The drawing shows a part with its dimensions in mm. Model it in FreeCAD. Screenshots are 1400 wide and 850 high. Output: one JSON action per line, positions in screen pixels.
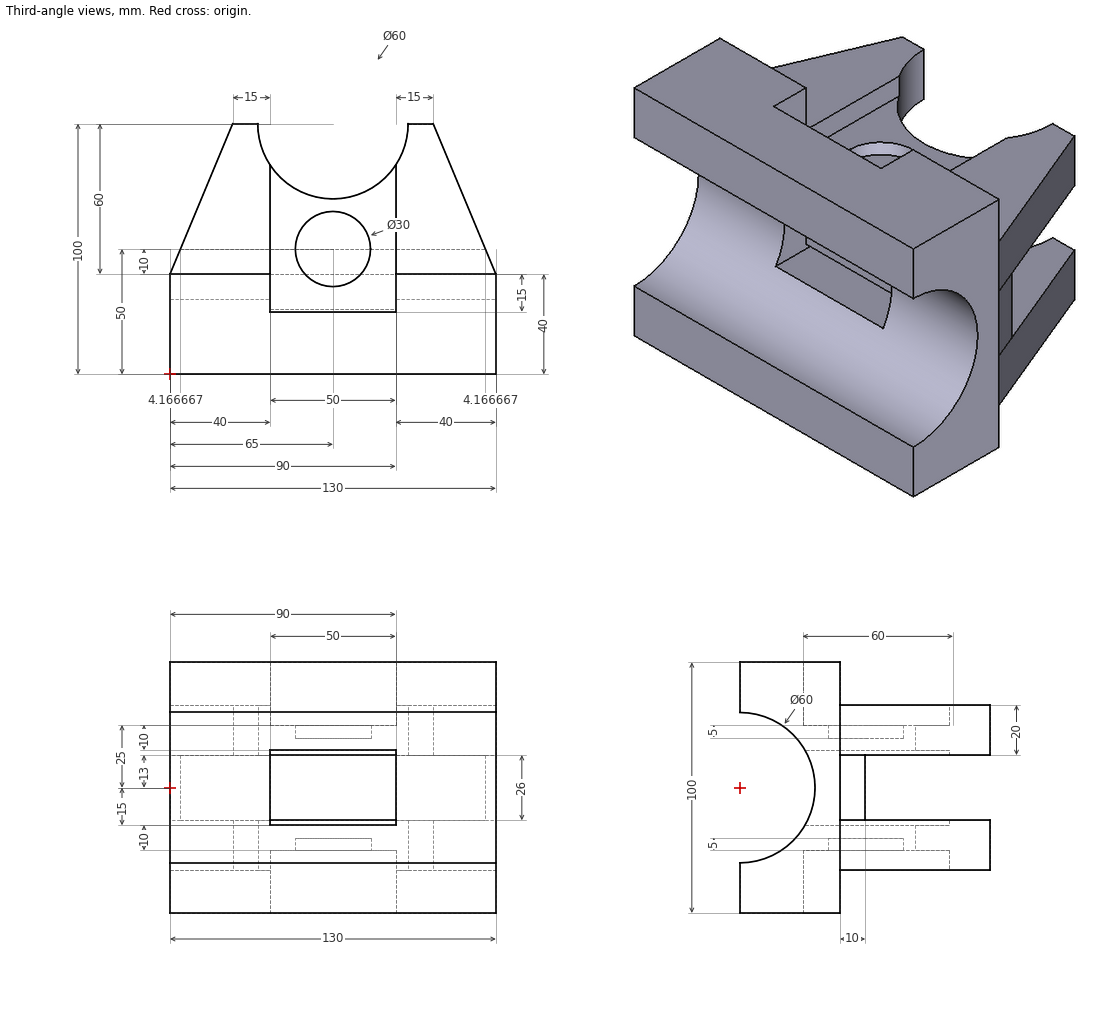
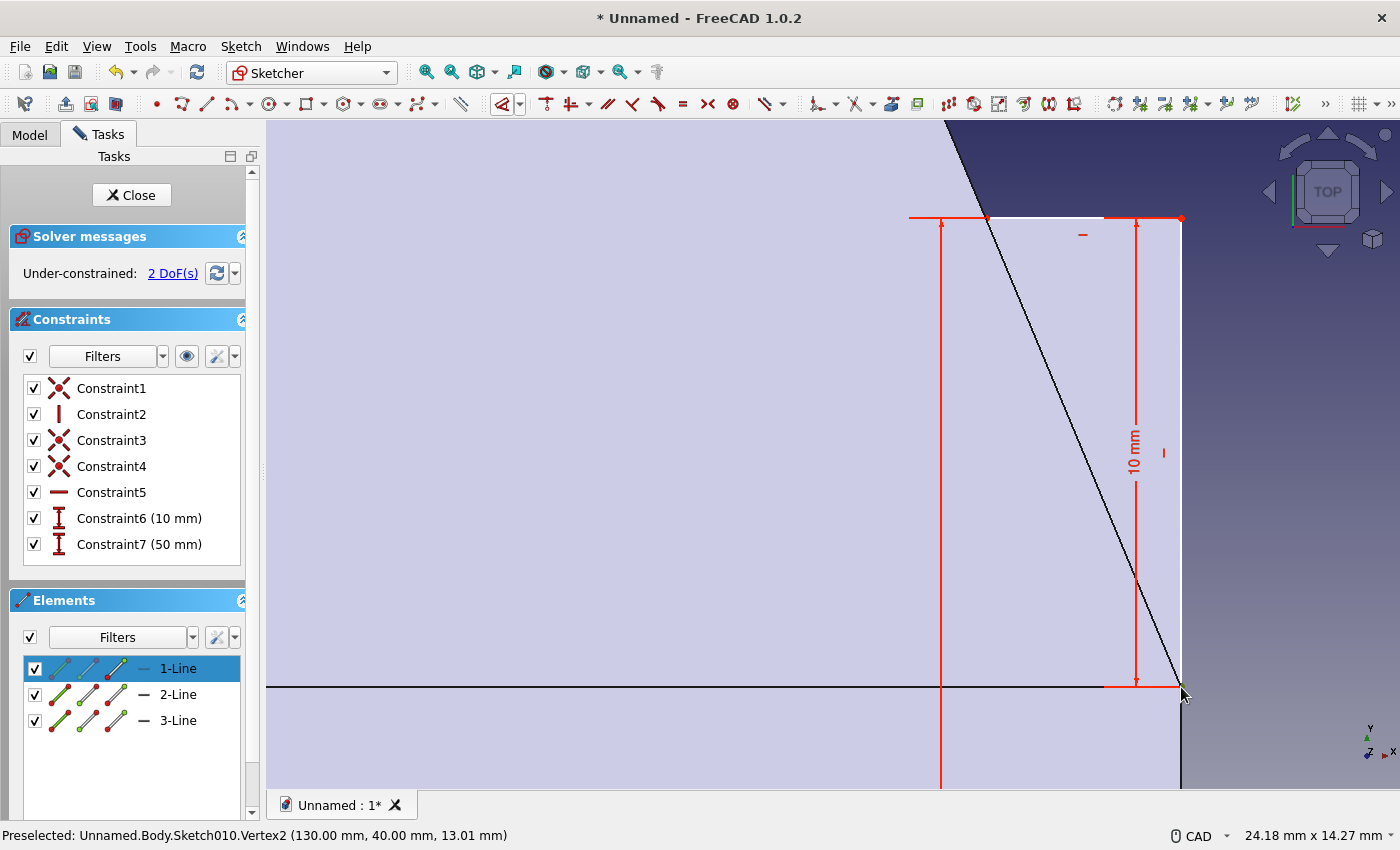
{"action": "left_click", "coordinate": [520, 104]}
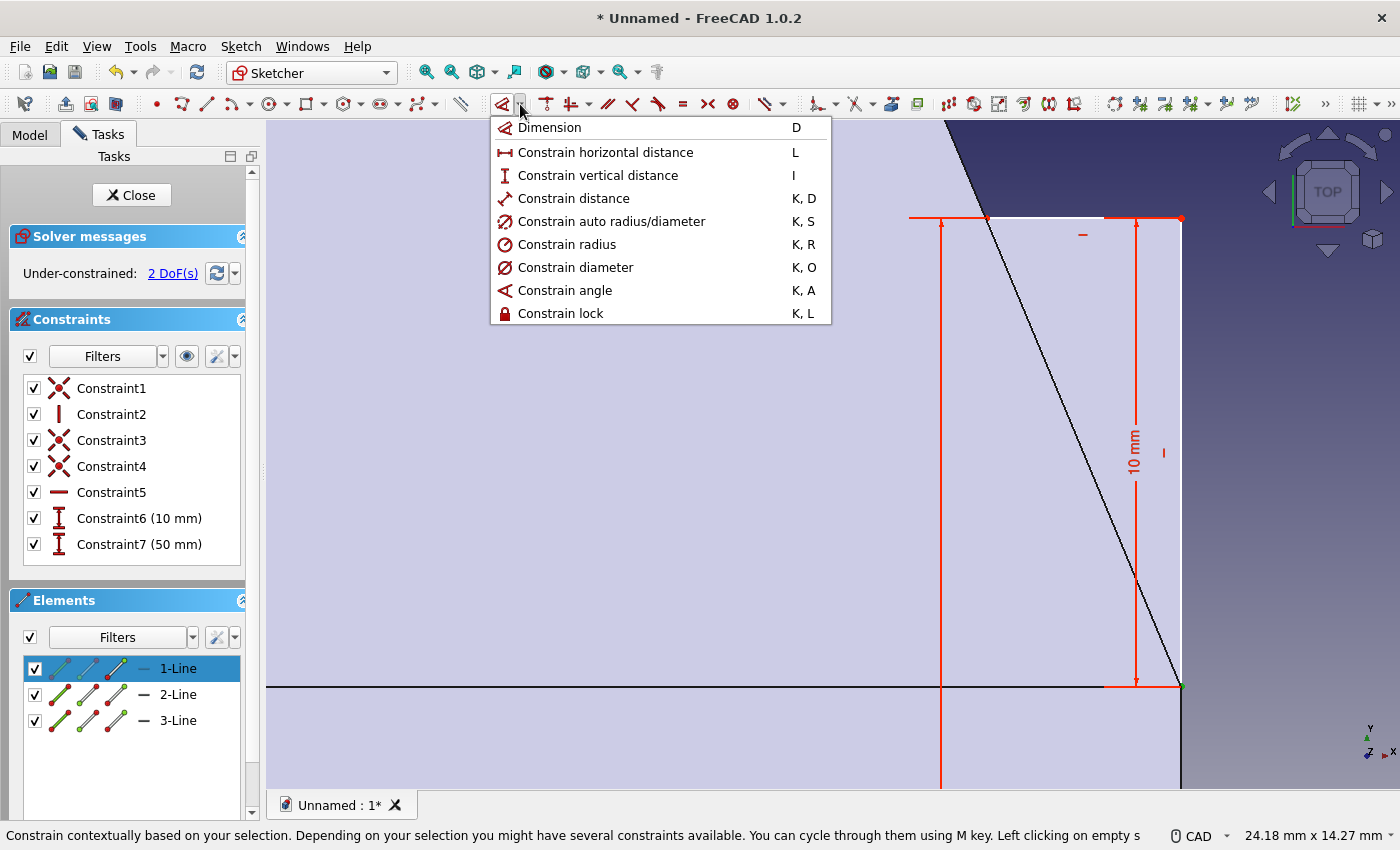
{"action": "left_click", "coordinate": [661, 152]}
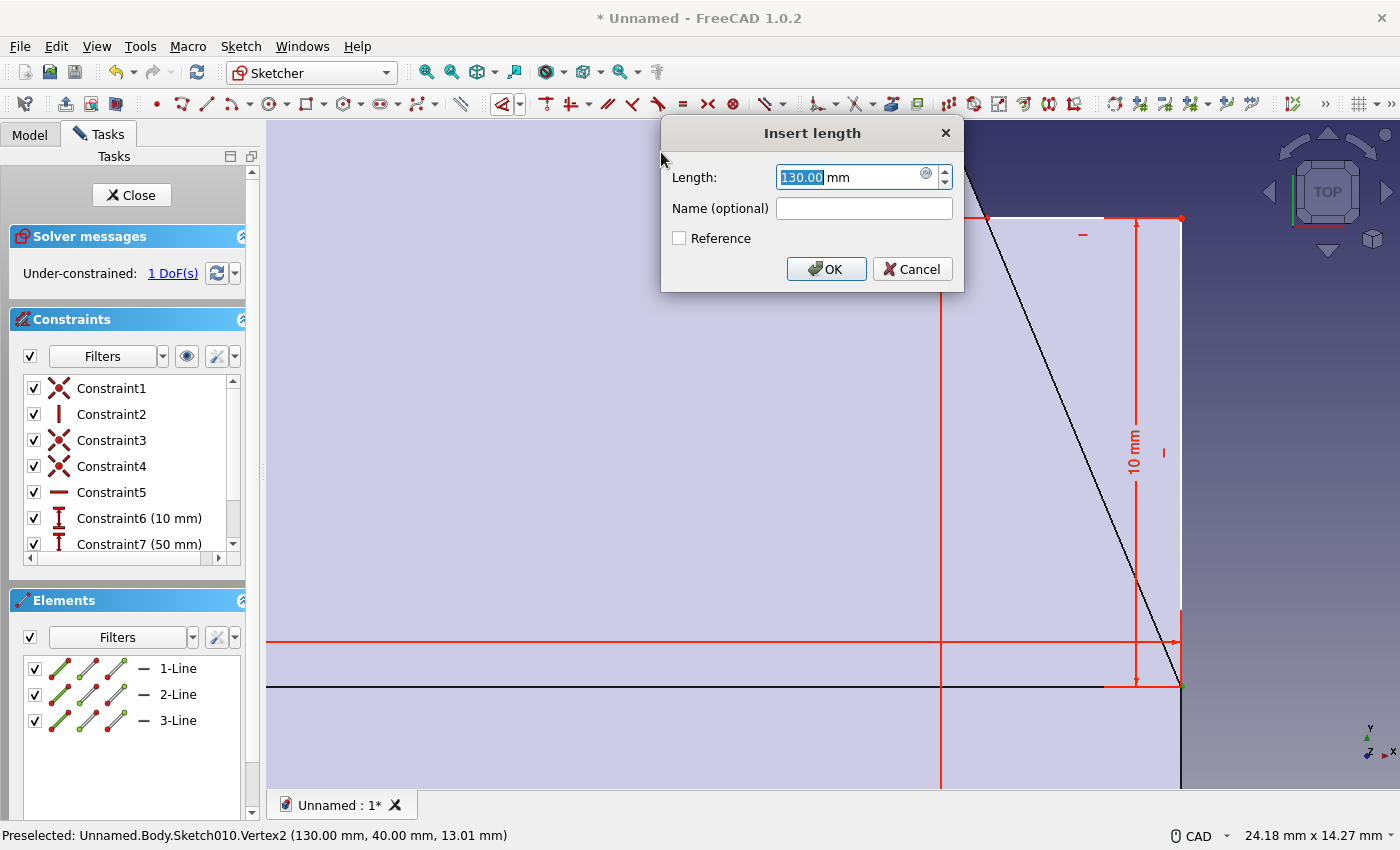
{"action": "type", "text": "130"}
{"action": "key", "text": "Return"}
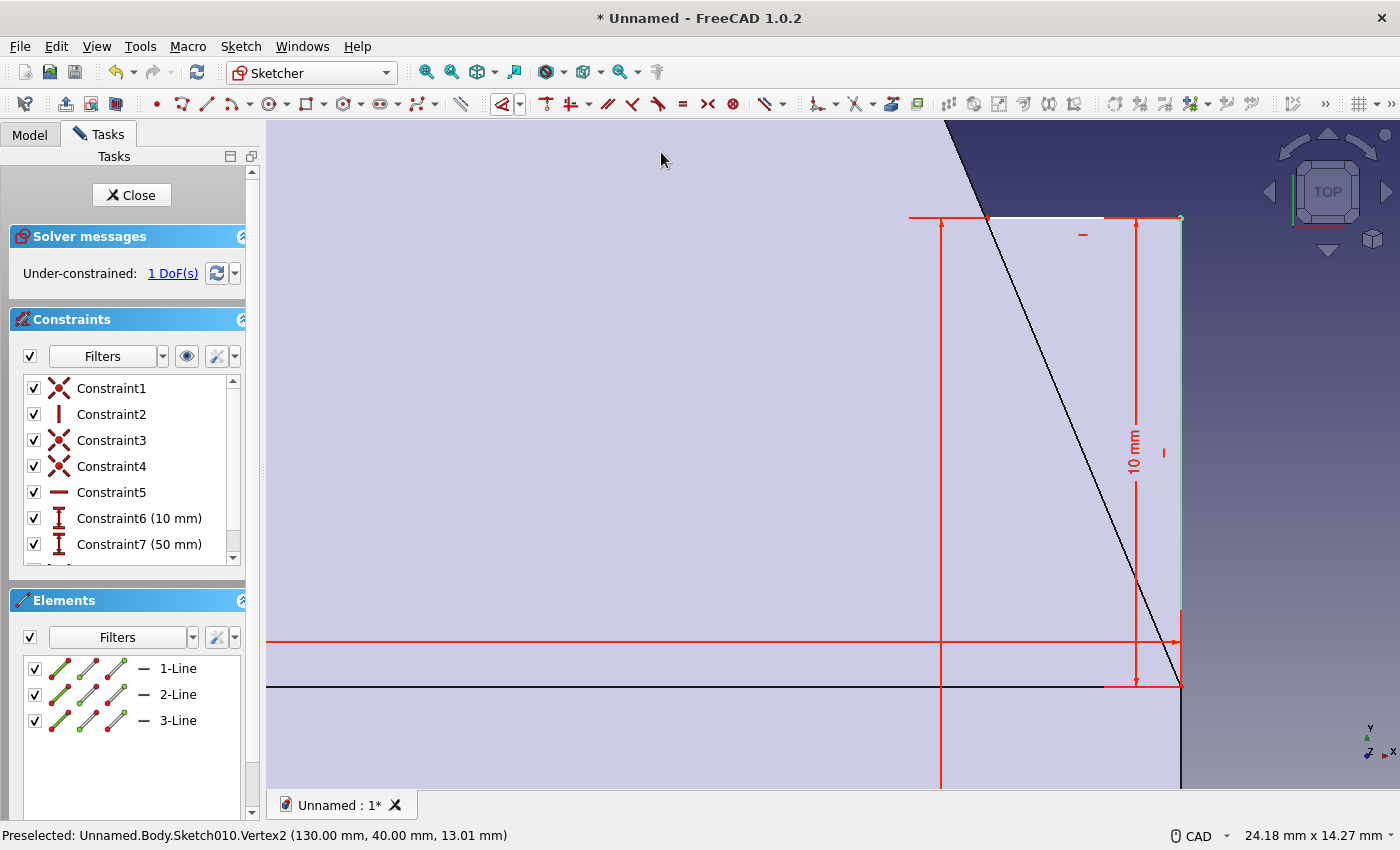
{"action": "left_click", "coordinate": [1122, 218]}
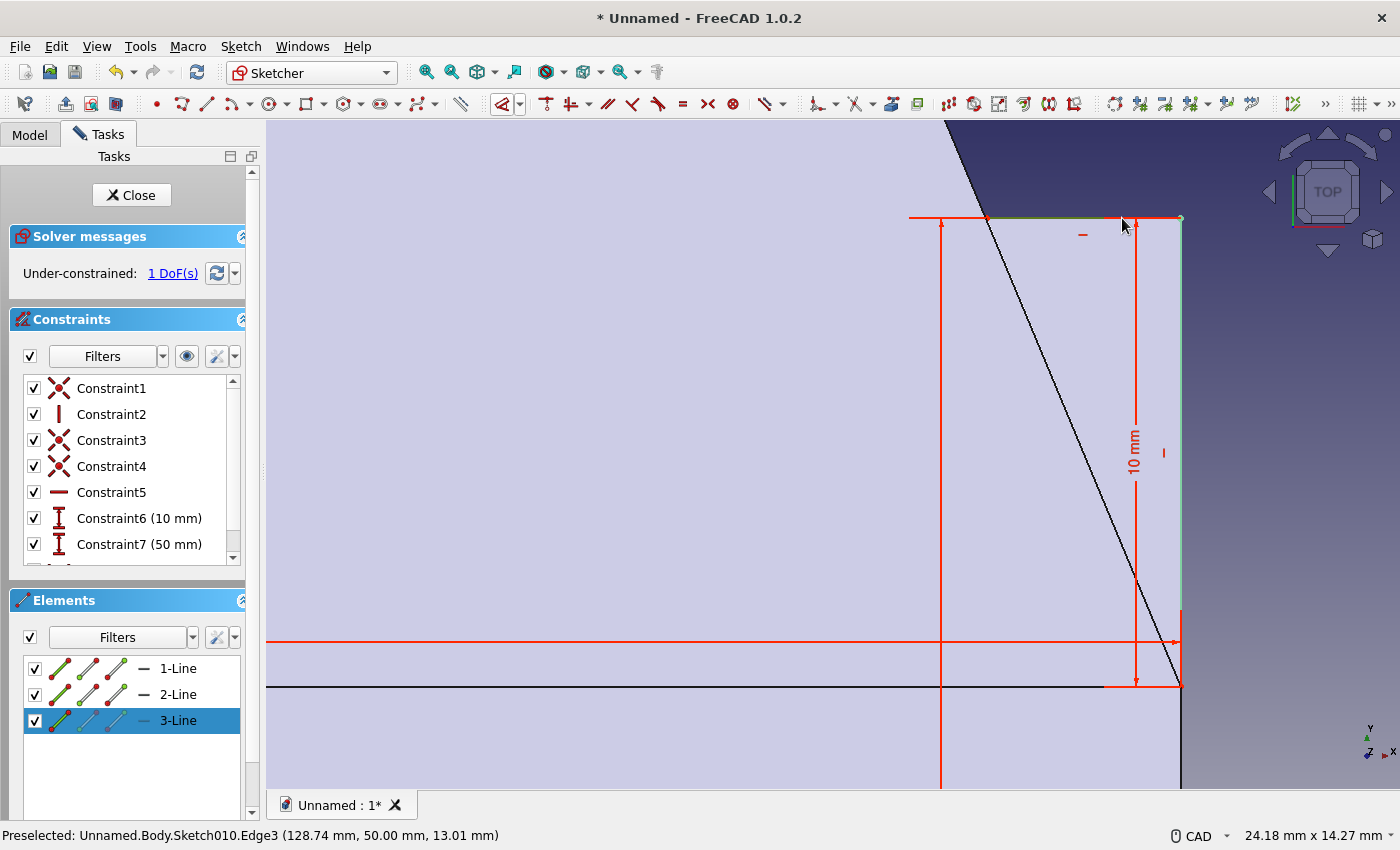
{"action": "key", "text": "l"}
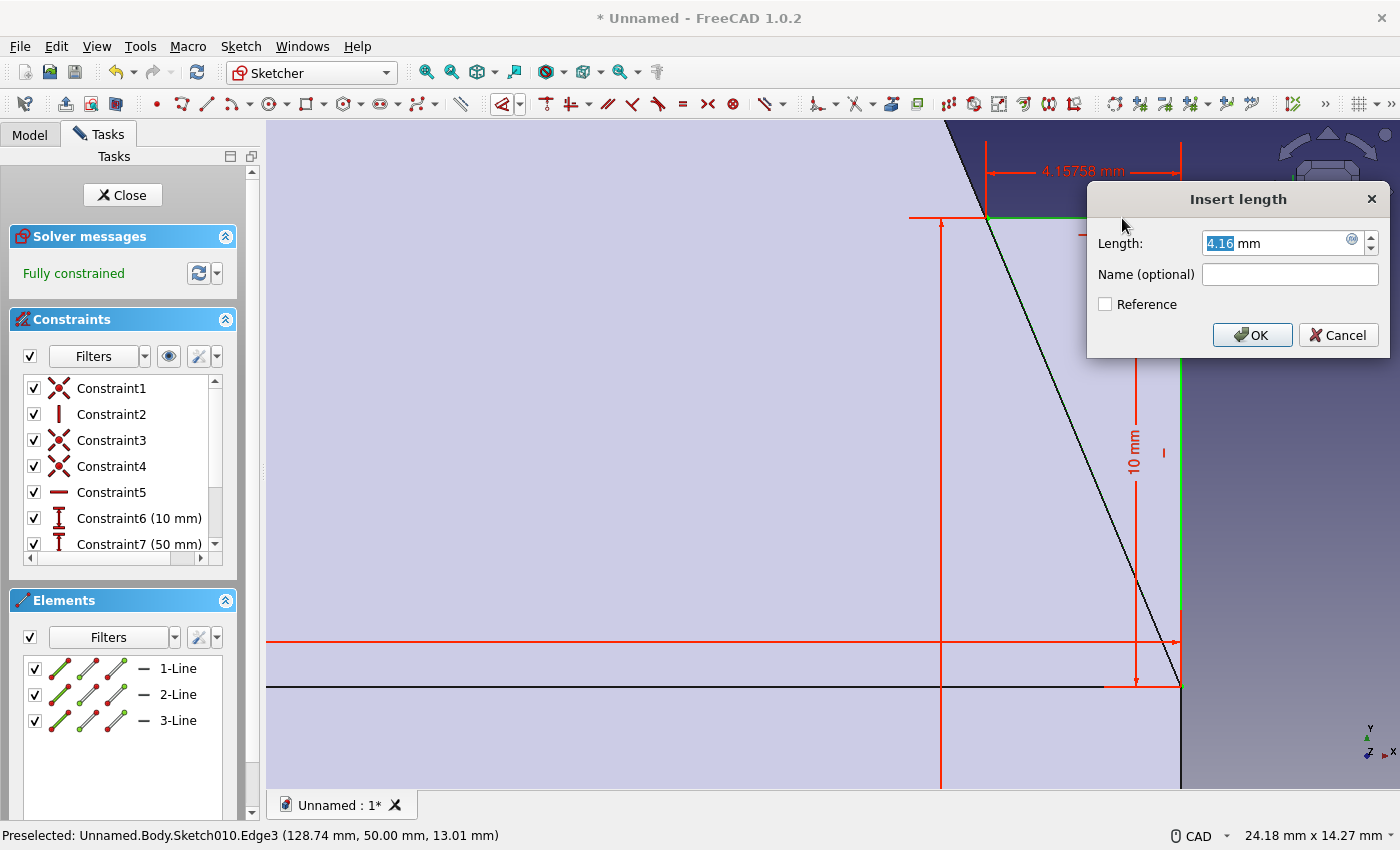
{"action": "type", "text": "4.166667"}
{"action": "key", "text": "Return"}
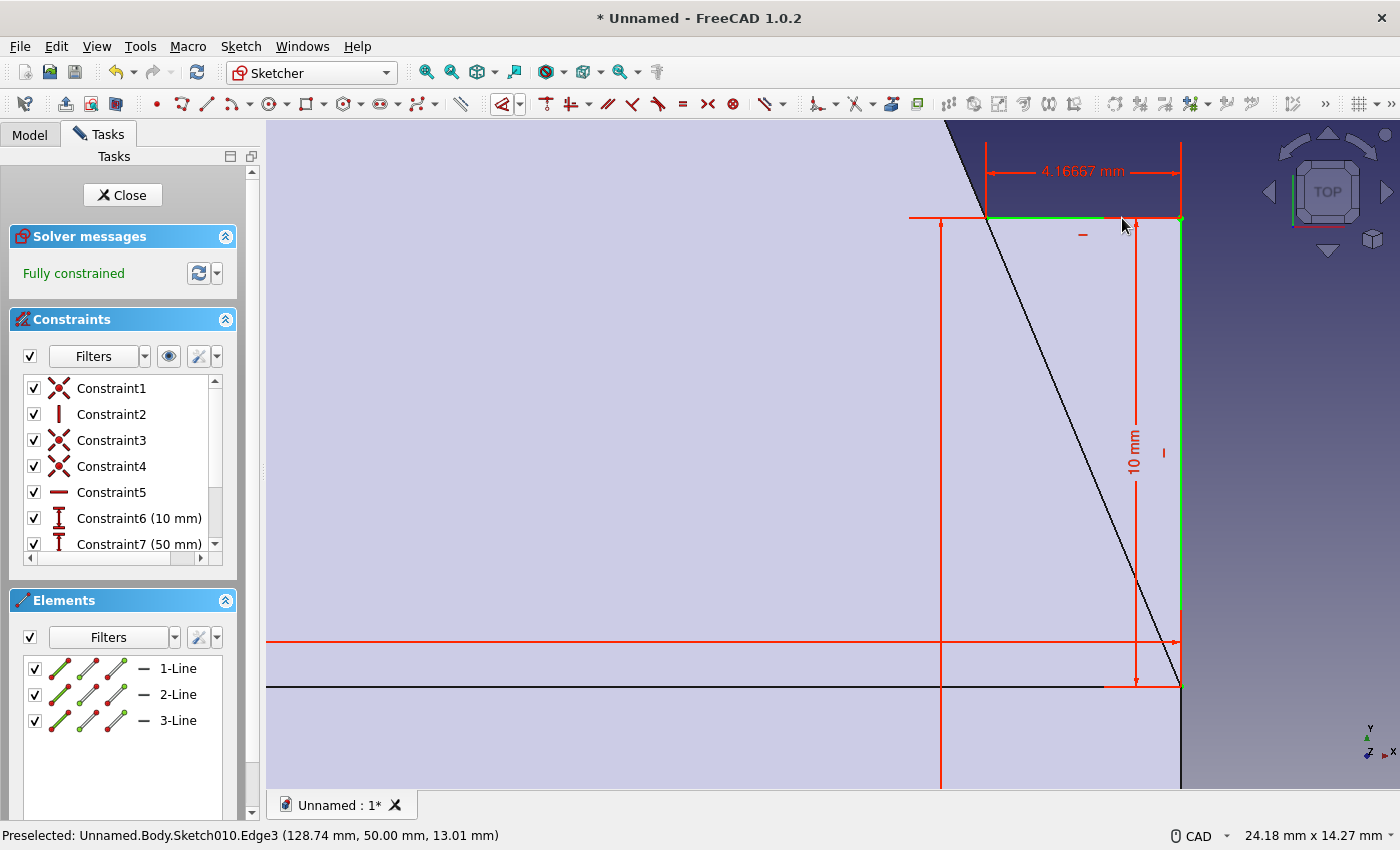
{"action": "left_click", "coordinate": [123, 195]}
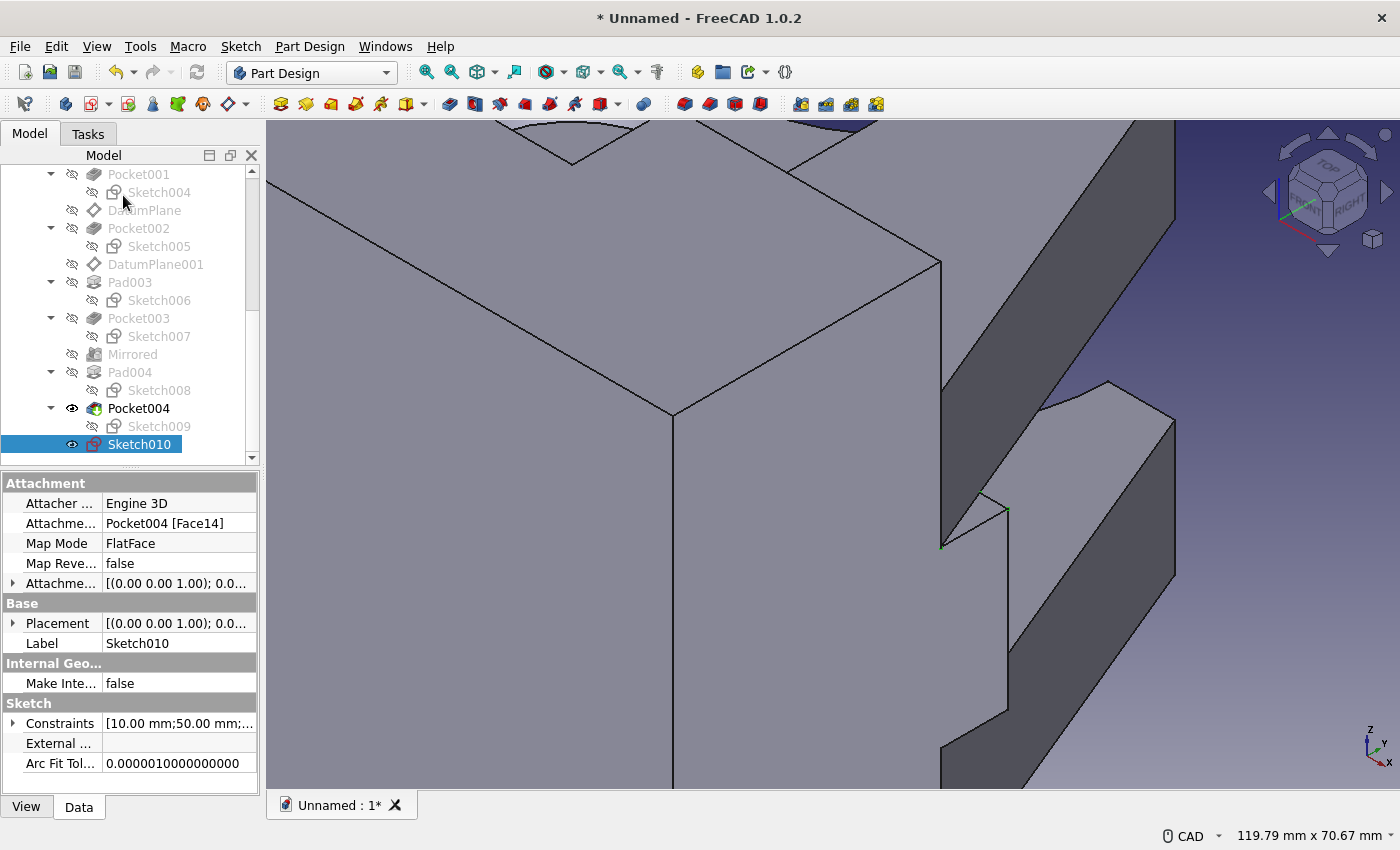
{"action": "left_click", "coordinate": [450, 104]}